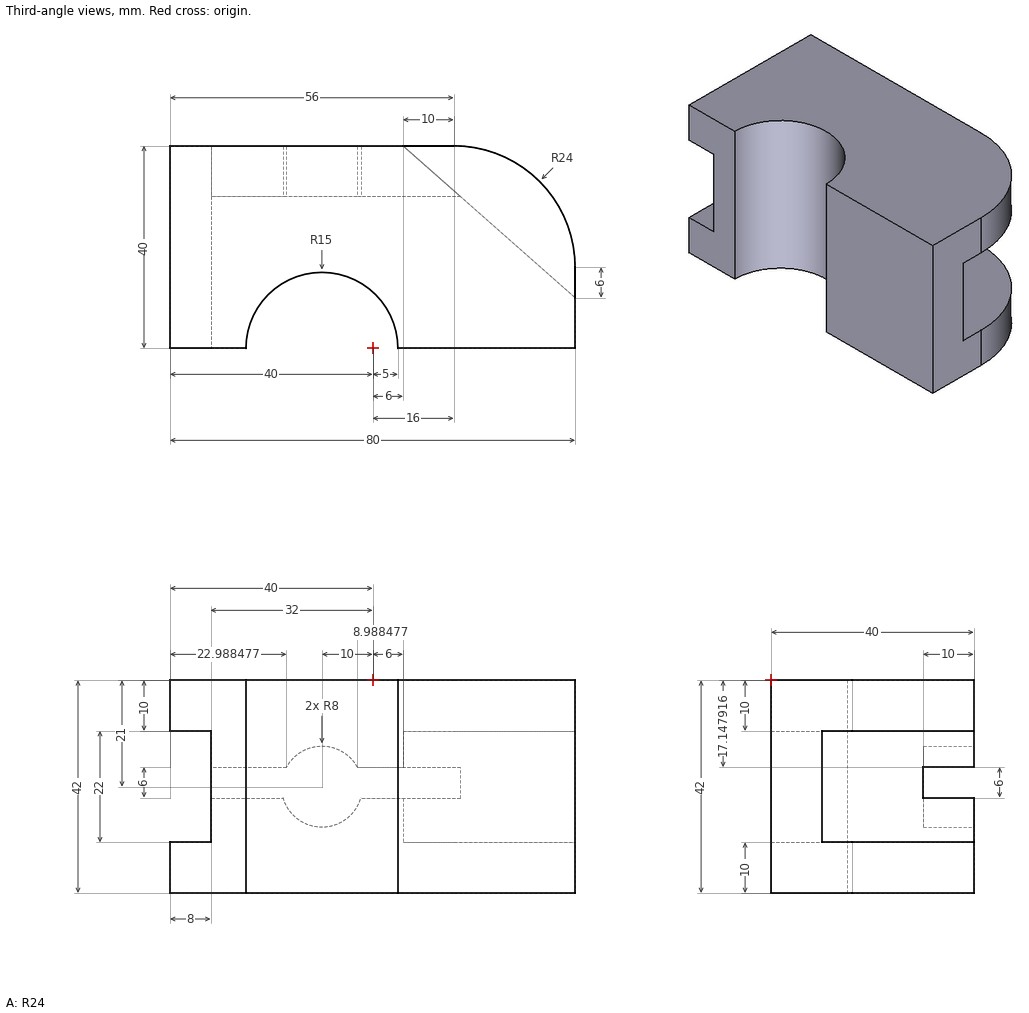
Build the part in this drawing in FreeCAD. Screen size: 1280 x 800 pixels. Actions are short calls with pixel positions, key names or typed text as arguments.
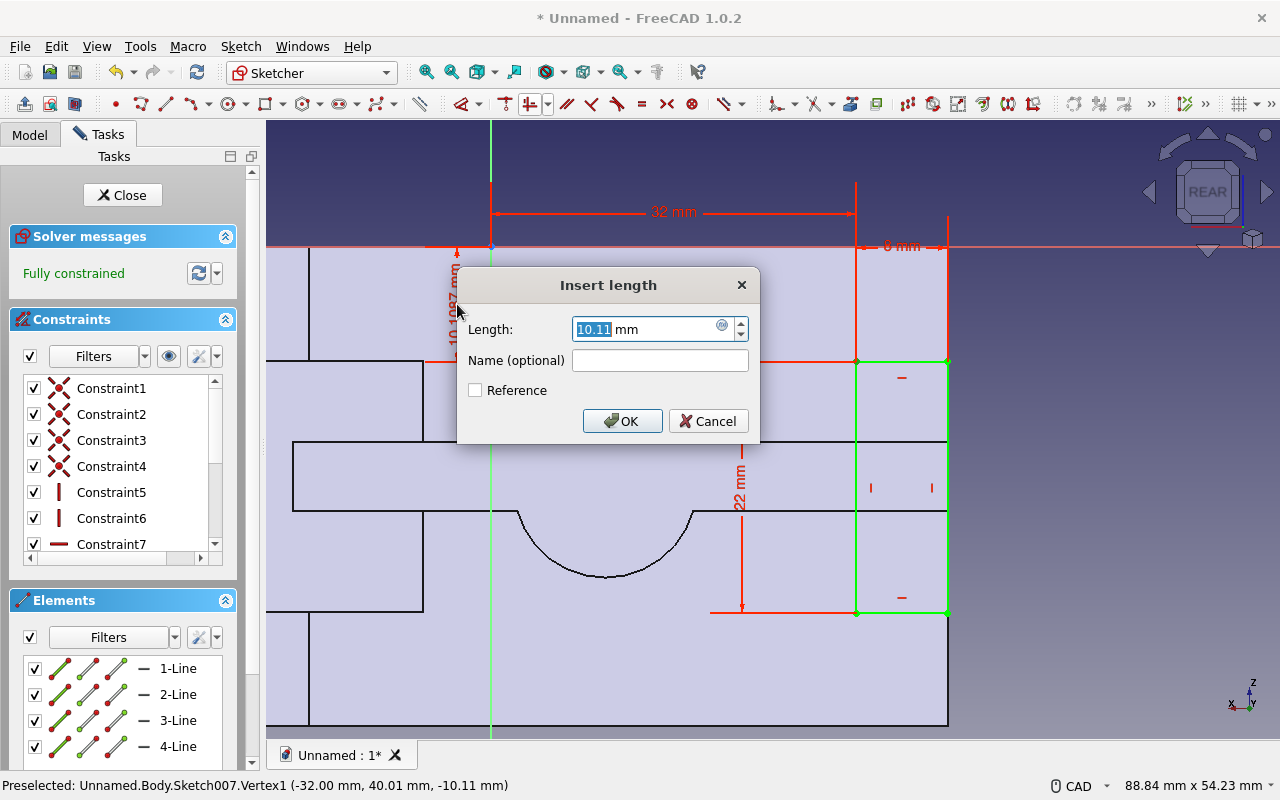
text(10)
key(Return)
key(Escape)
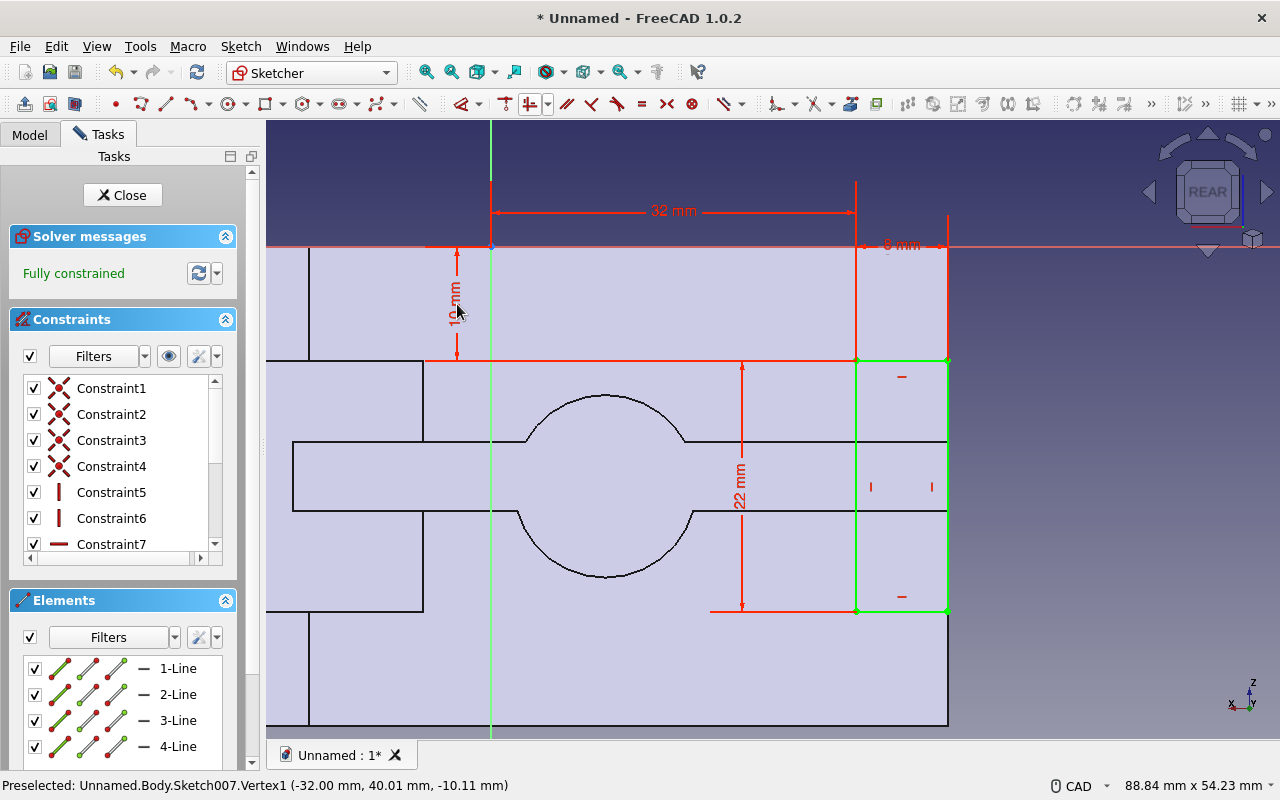
click(123, 195)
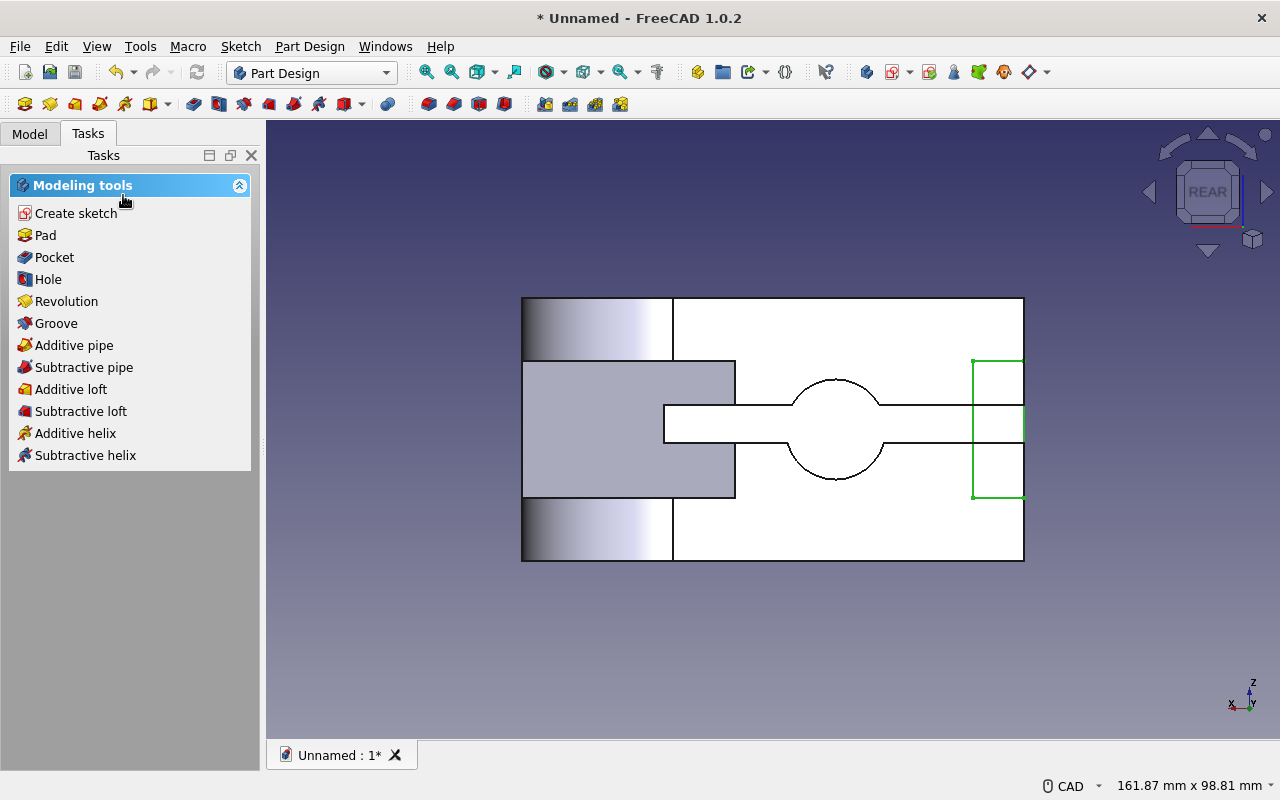
click(194, 104)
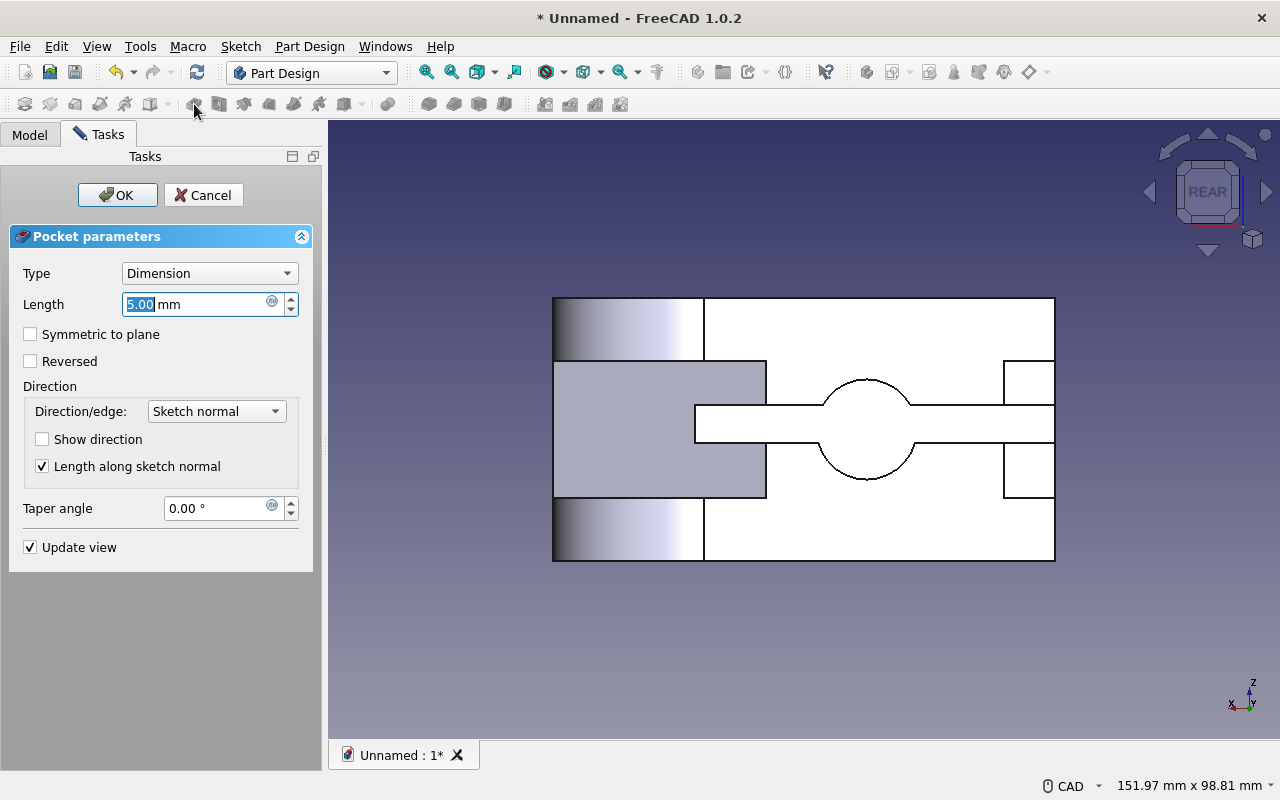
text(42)
key(Tab)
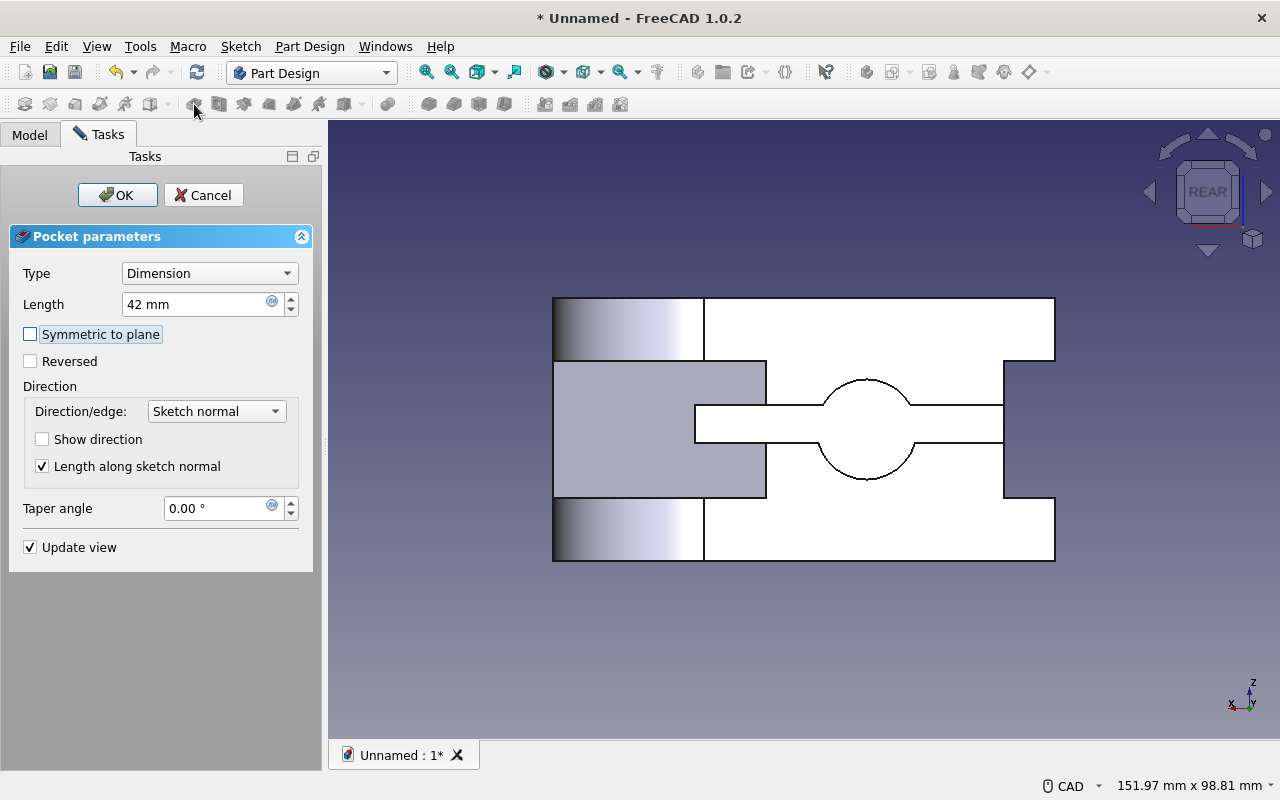
click(118, 195)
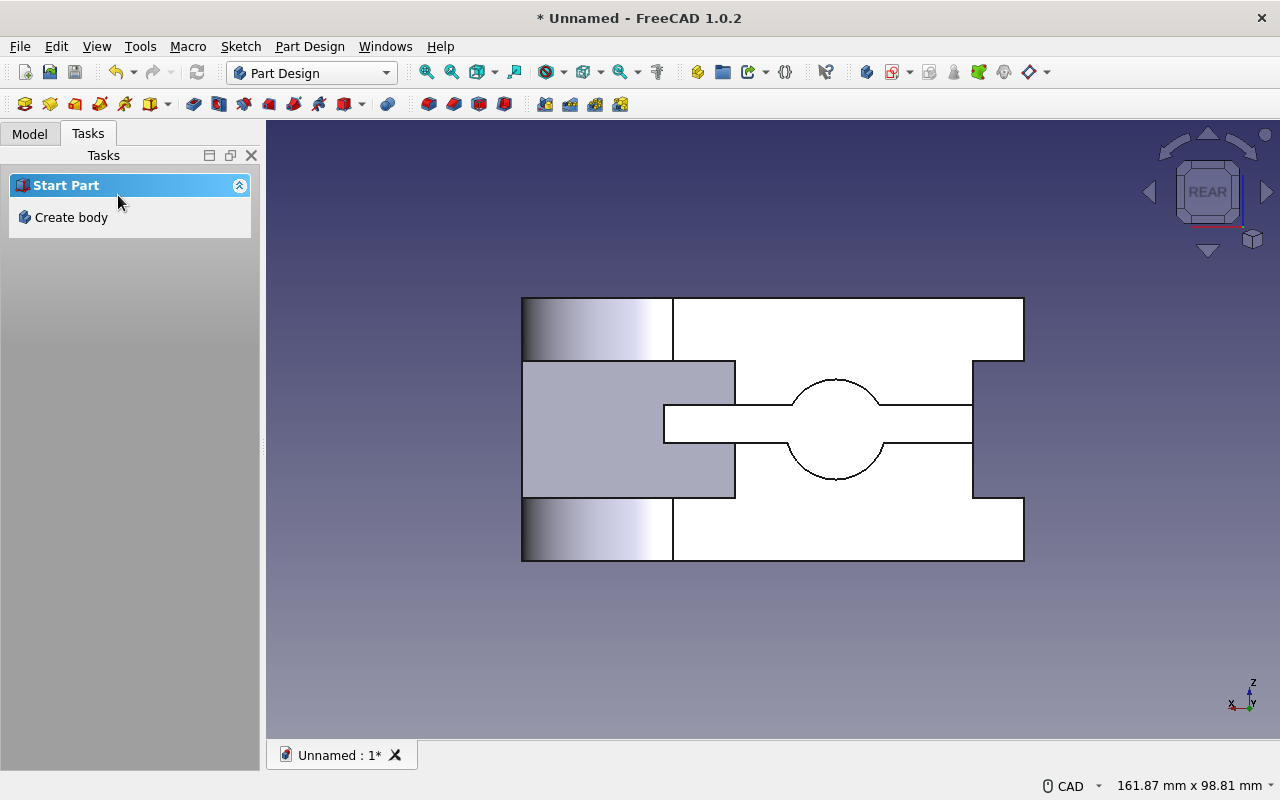
key(0)